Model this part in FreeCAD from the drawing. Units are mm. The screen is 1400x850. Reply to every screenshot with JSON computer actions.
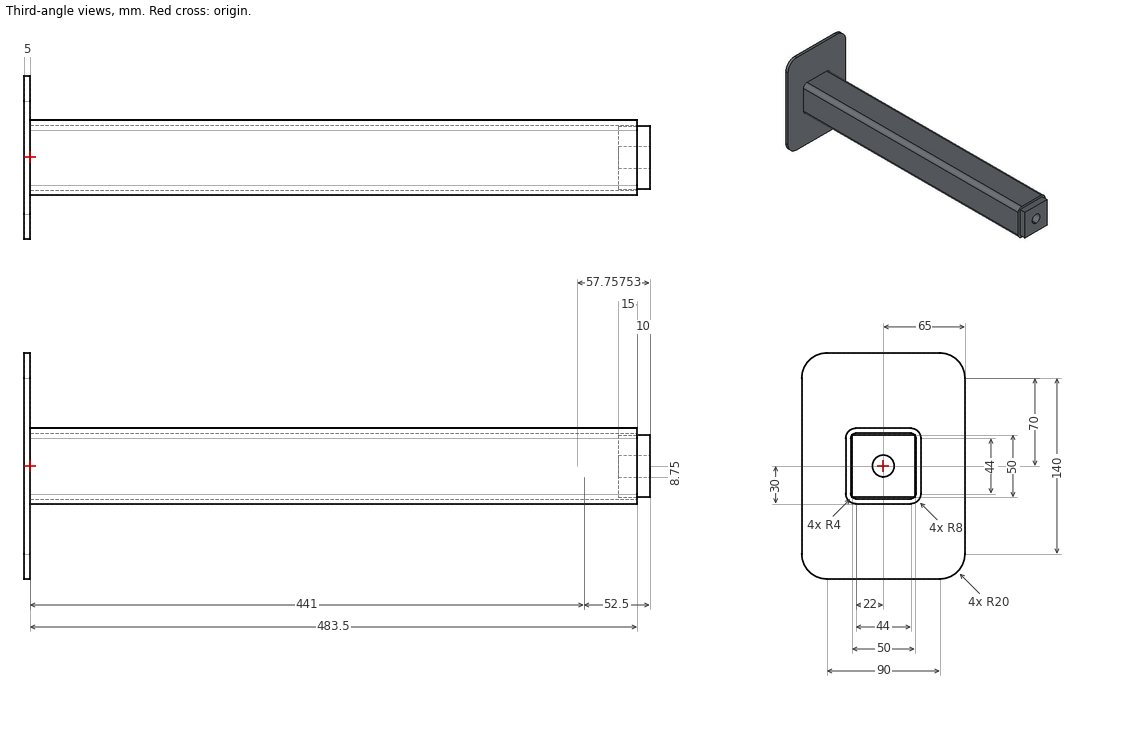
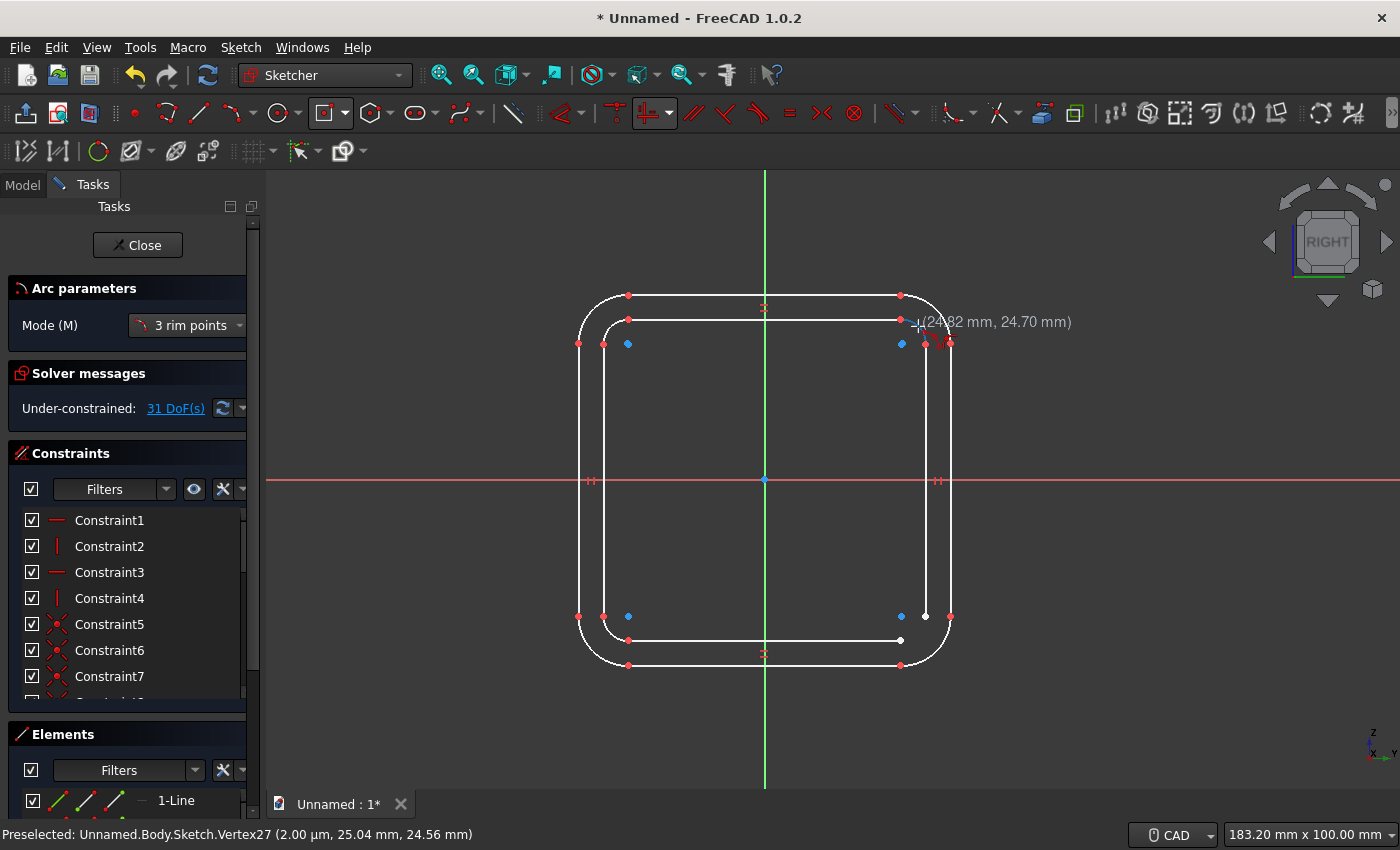
{"action": "left_click", "coordinate": [926, 617]}
{"action": "left_click", "coordinate": [901, 641]}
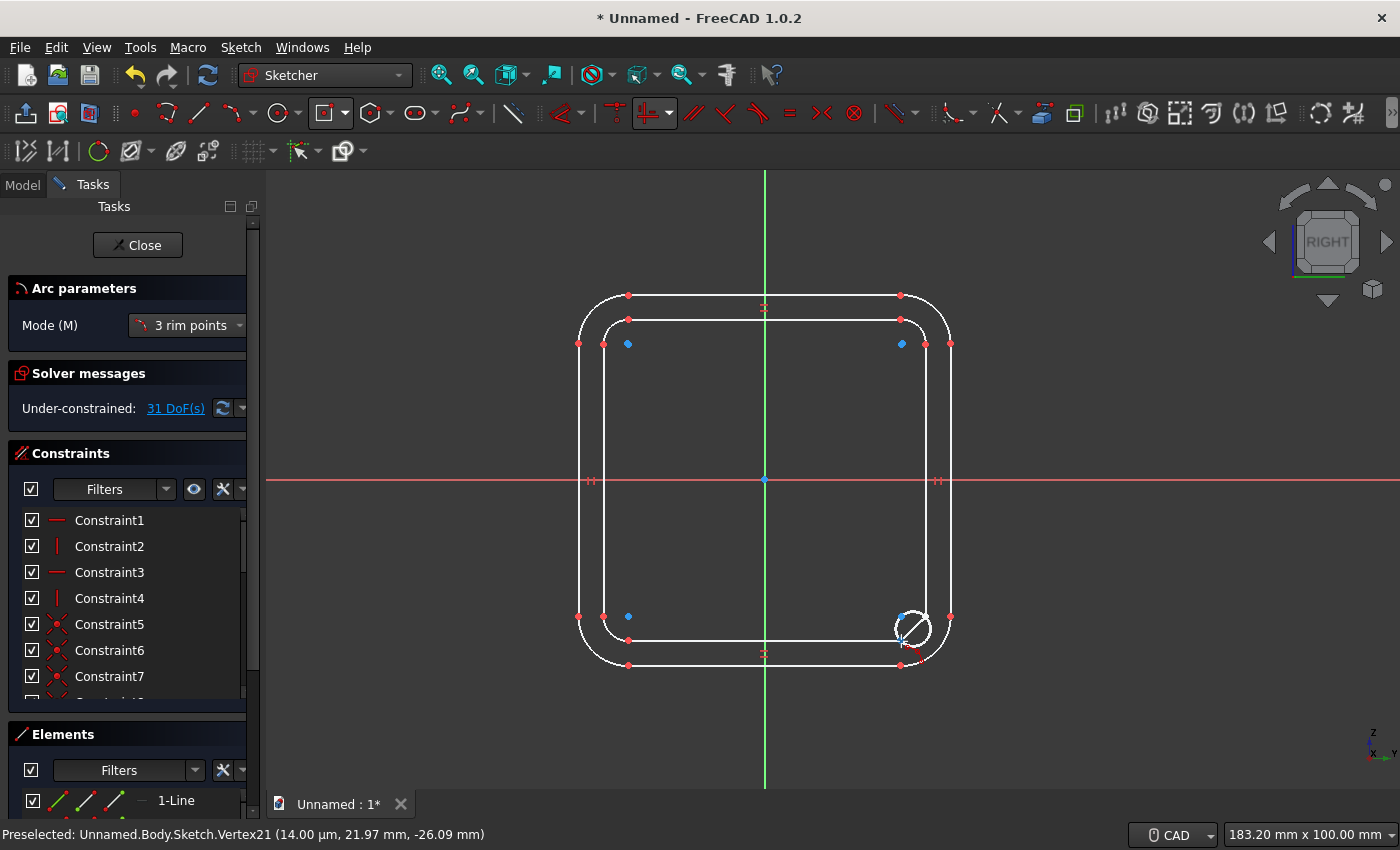
{"action": "scroll", "coordinate": [918, 633], "scroll_direction": "up", "scroll_amount": 4}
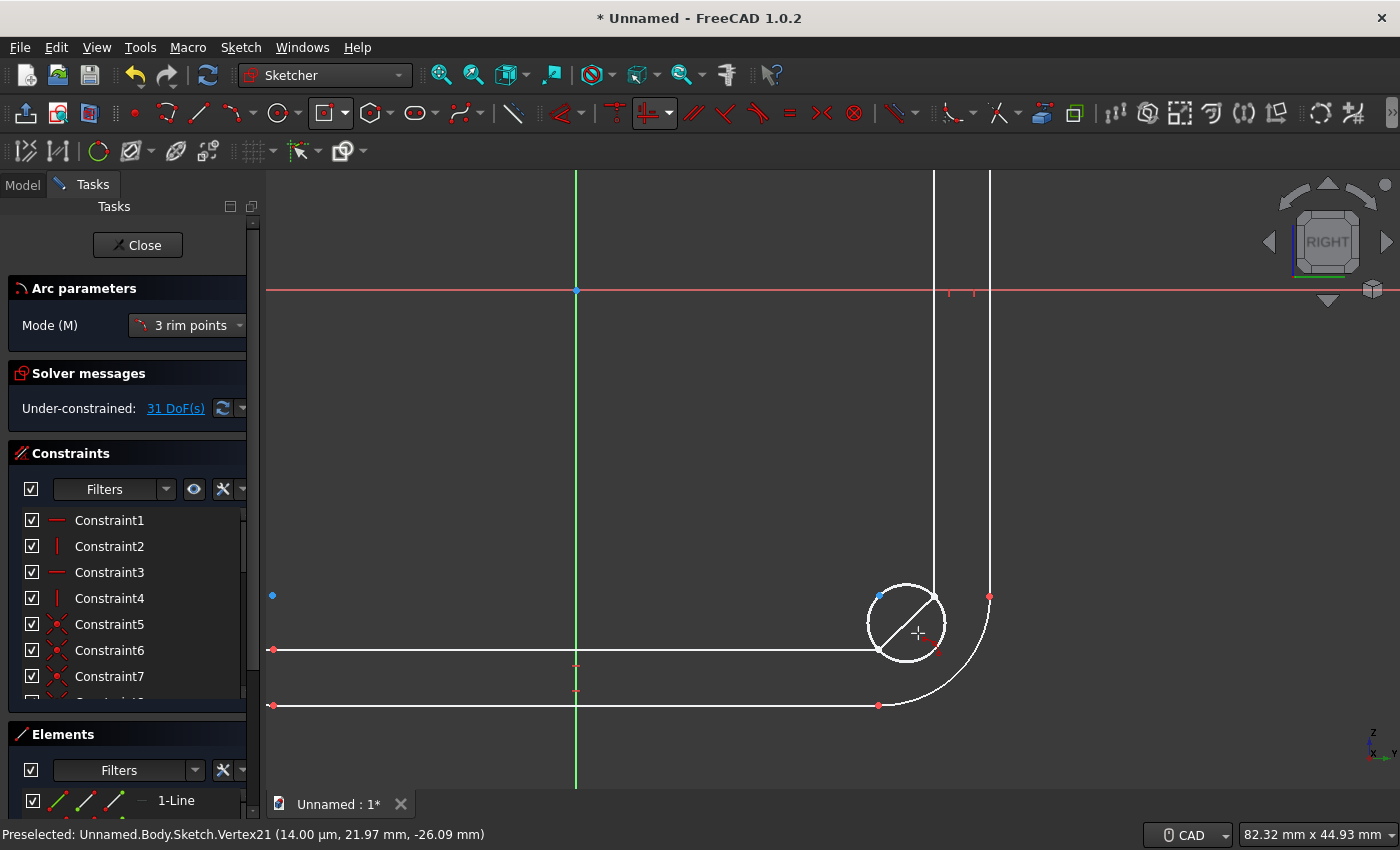
{"action": "left_click", "coordinate": [918, 633]}
{"action": "key", "text": "Escape"}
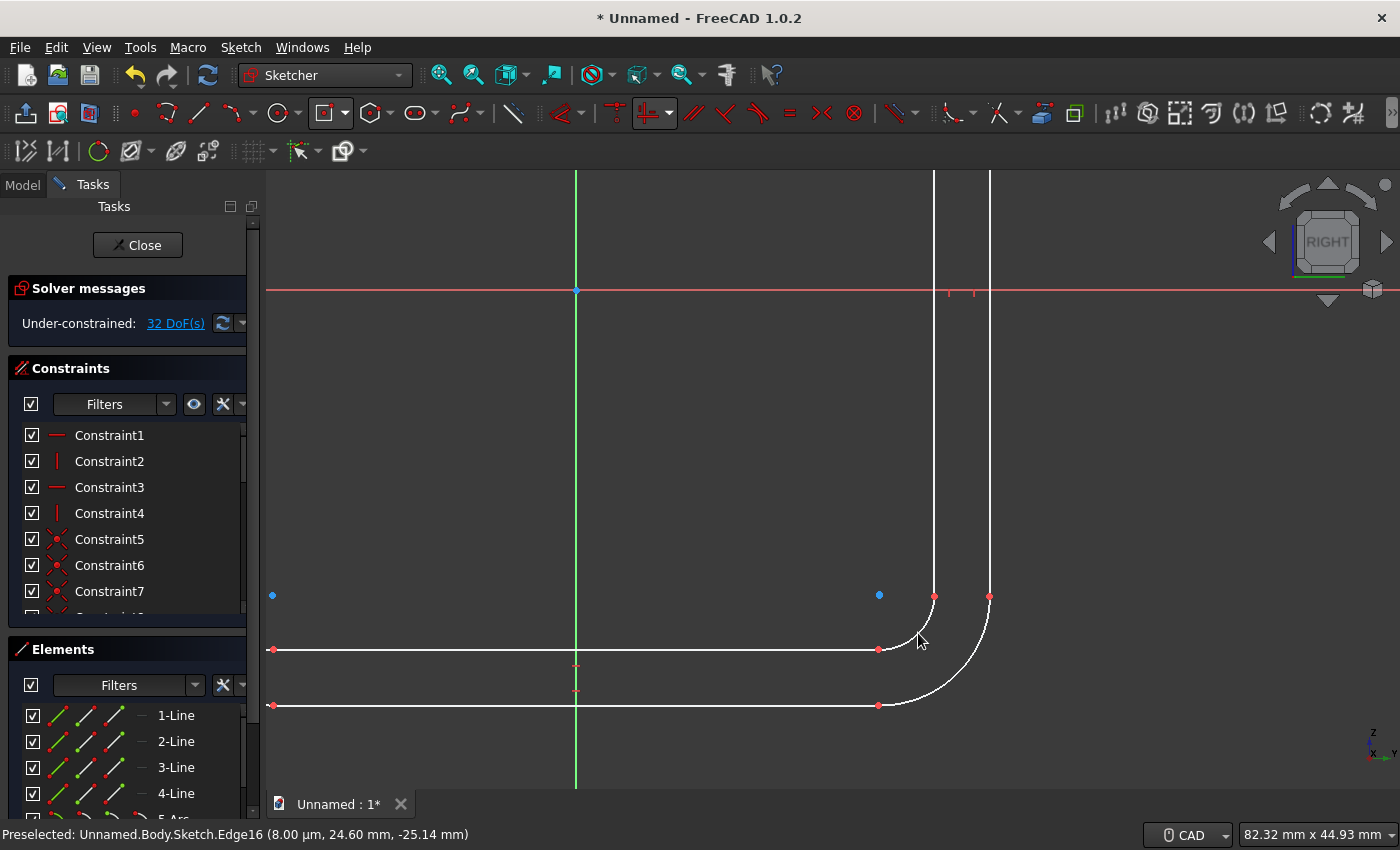
{"action": "left_click", "coordinate": [455, 706]}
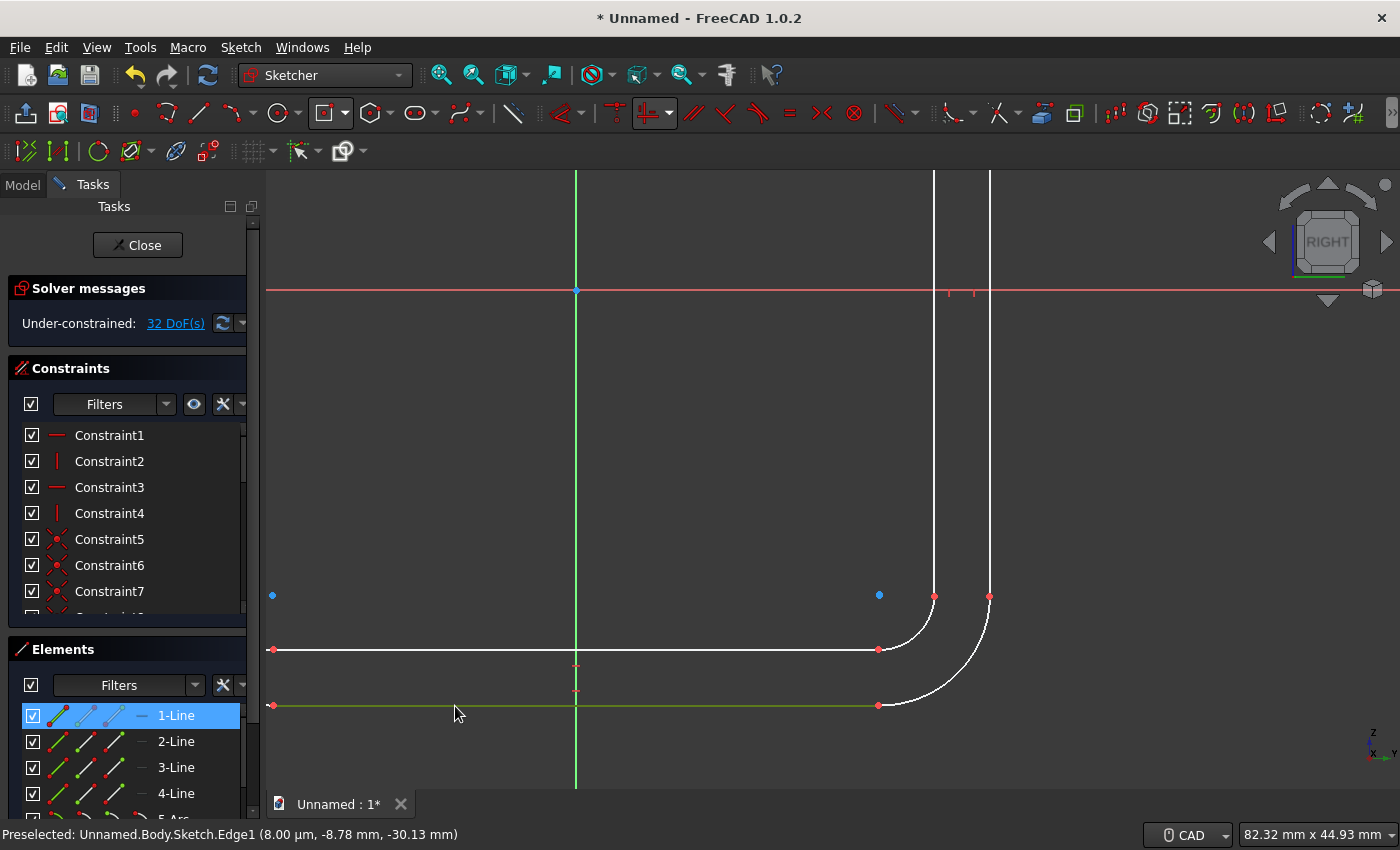
{"action": "left_click", "coordinate": [929, 694]}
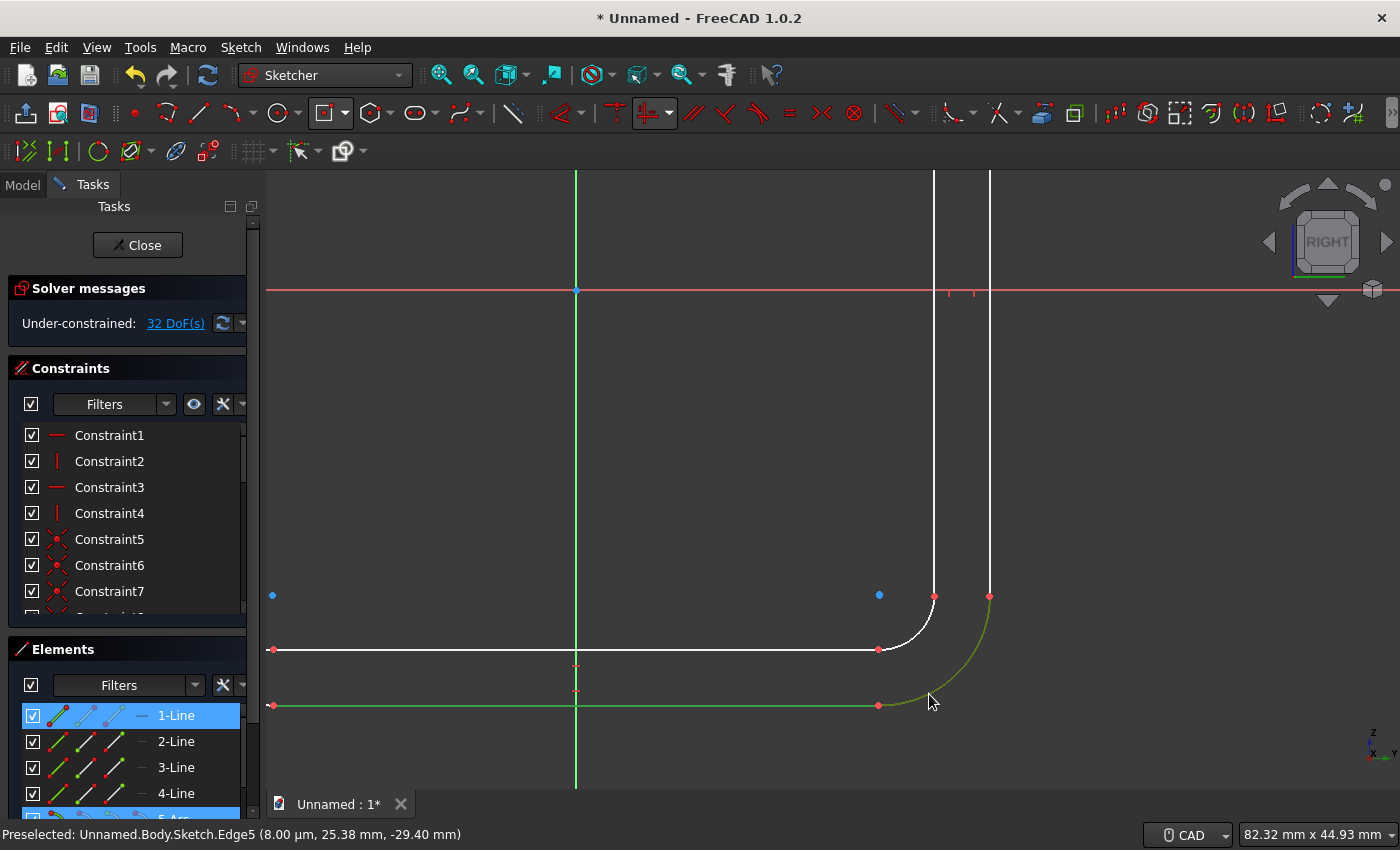
{"action": "key", "text": "t"}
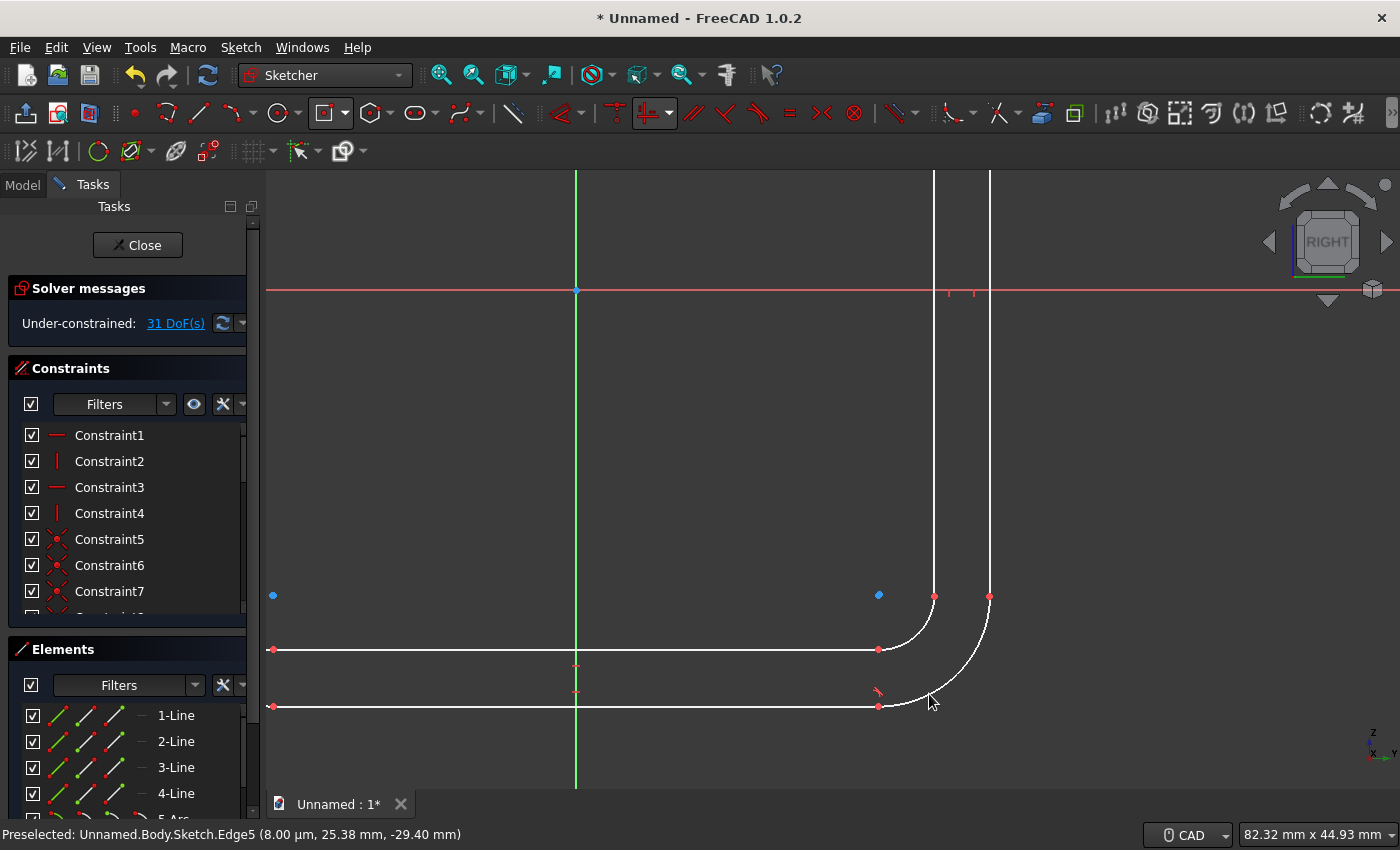
{"action": "left_click", "coordinate": [455, 707]}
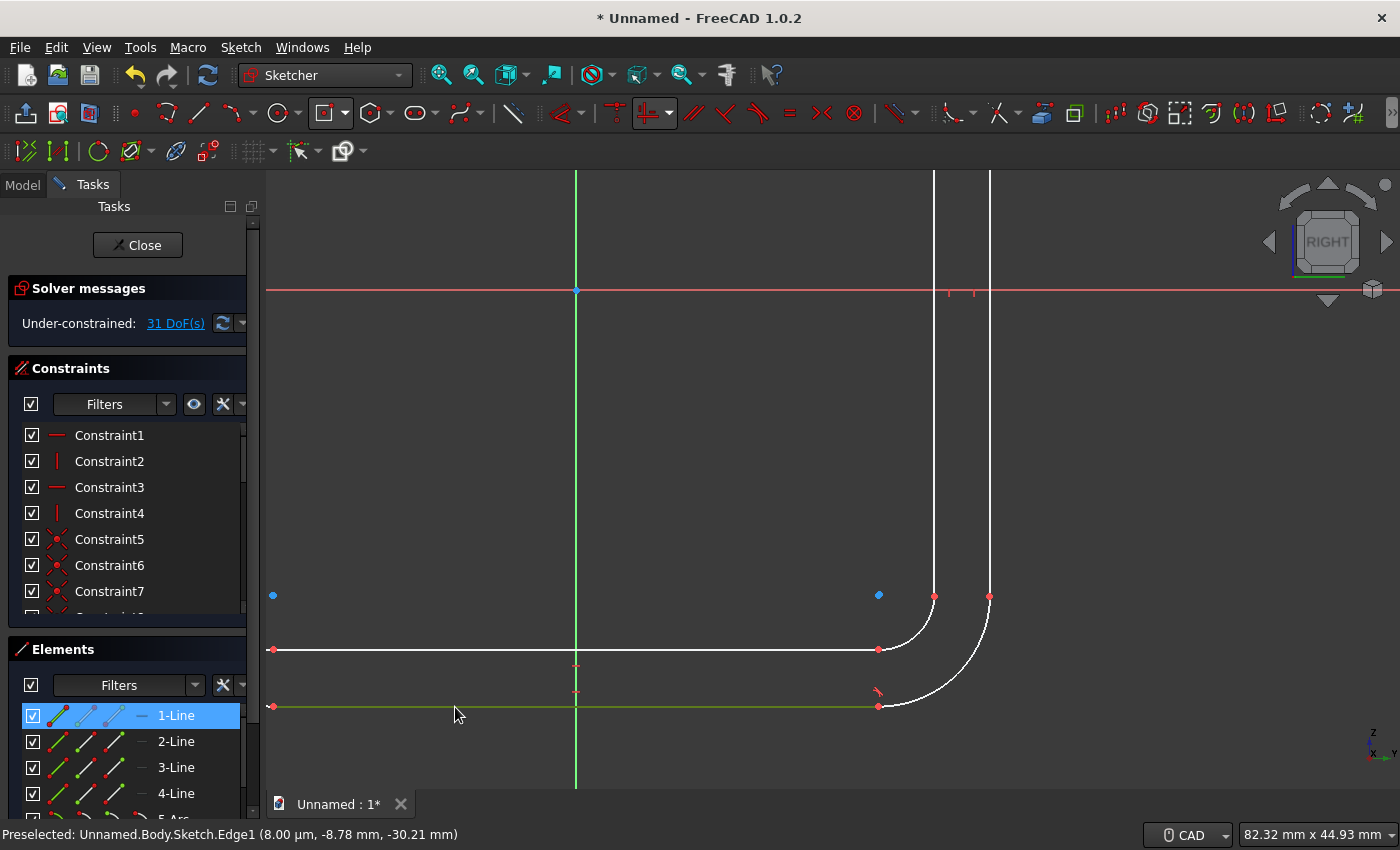
{"action": "scroll", "coordinate": [918, 634], "scroll_direction": "down", "scroll_amount": 4}